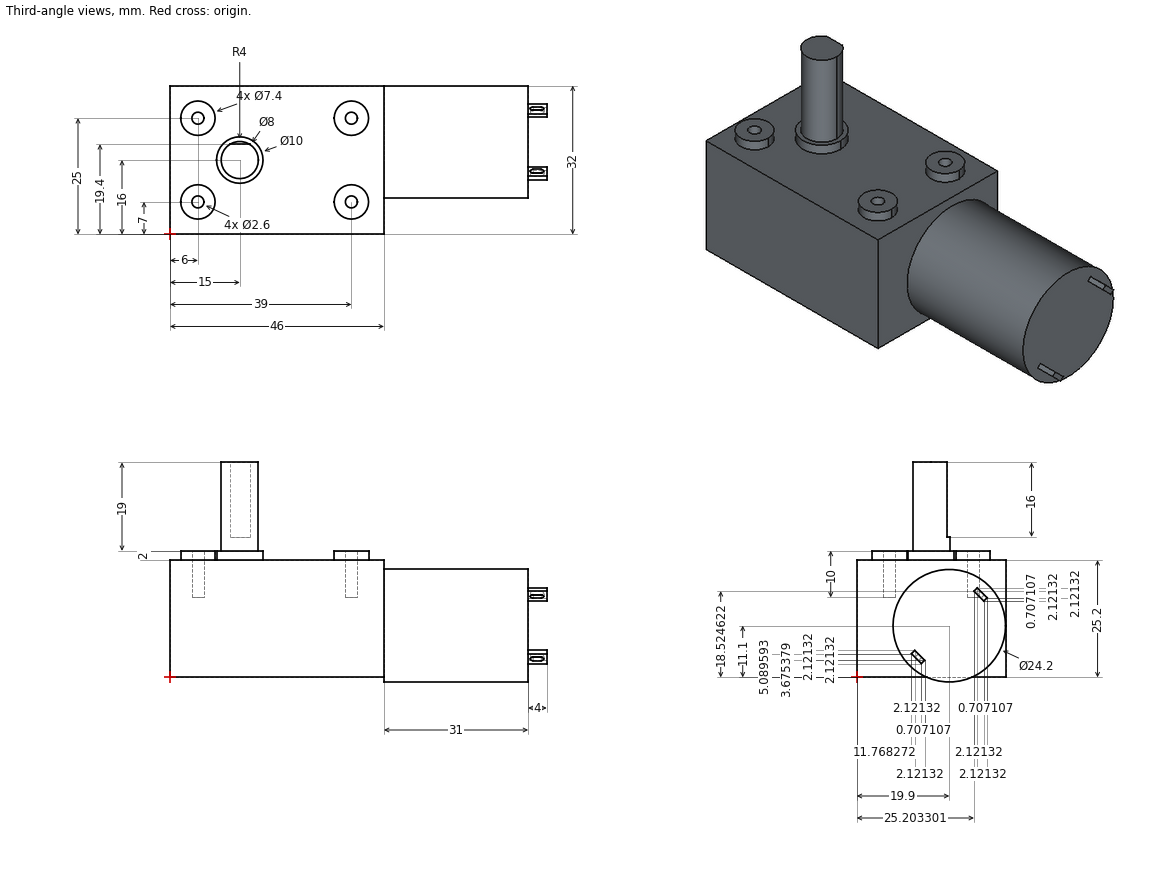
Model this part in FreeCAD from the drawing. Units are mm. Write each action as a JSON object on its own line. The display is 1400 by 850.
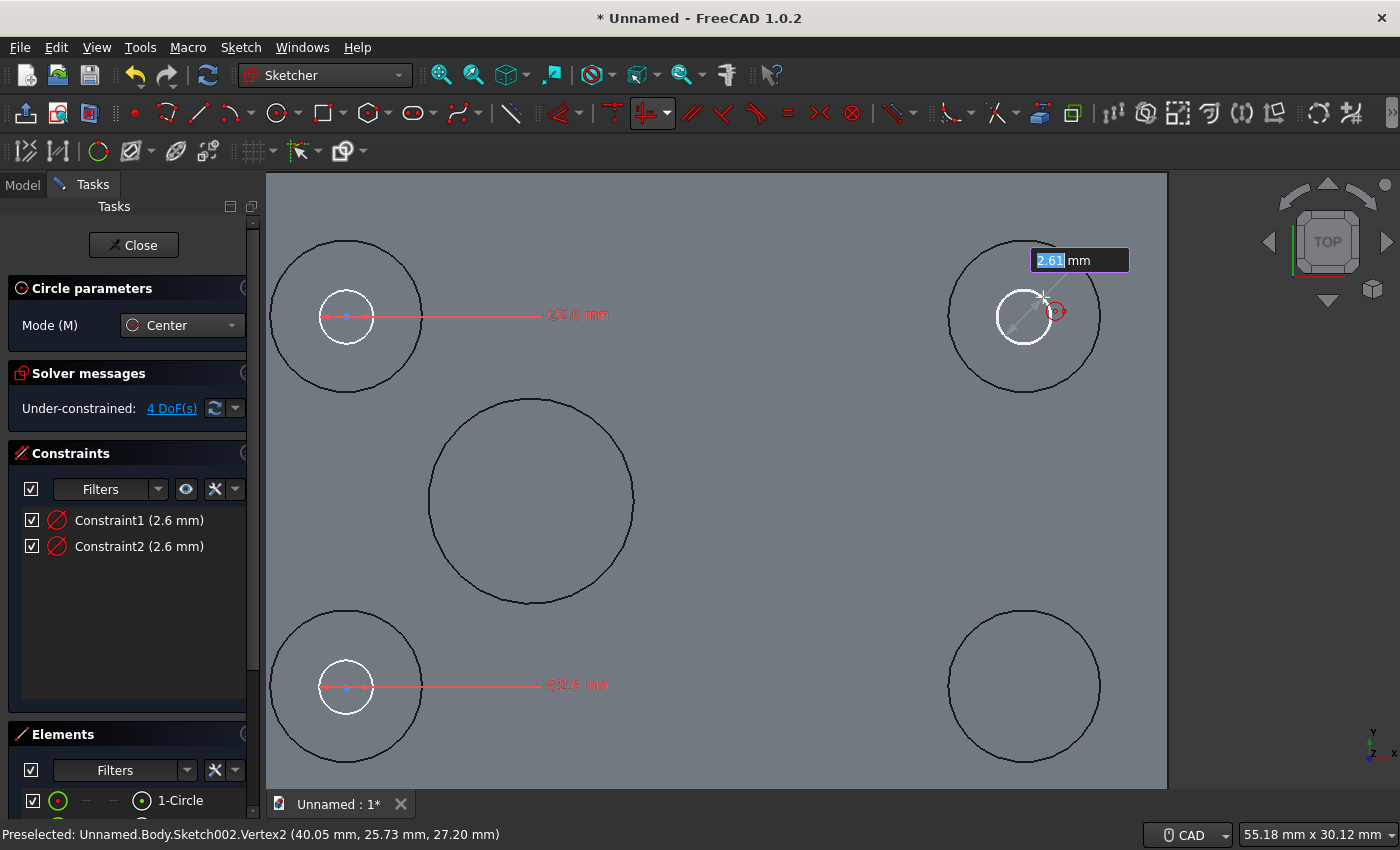
{"action": "type", "text": "2.6"}
{"action": "key", "text": "Return"}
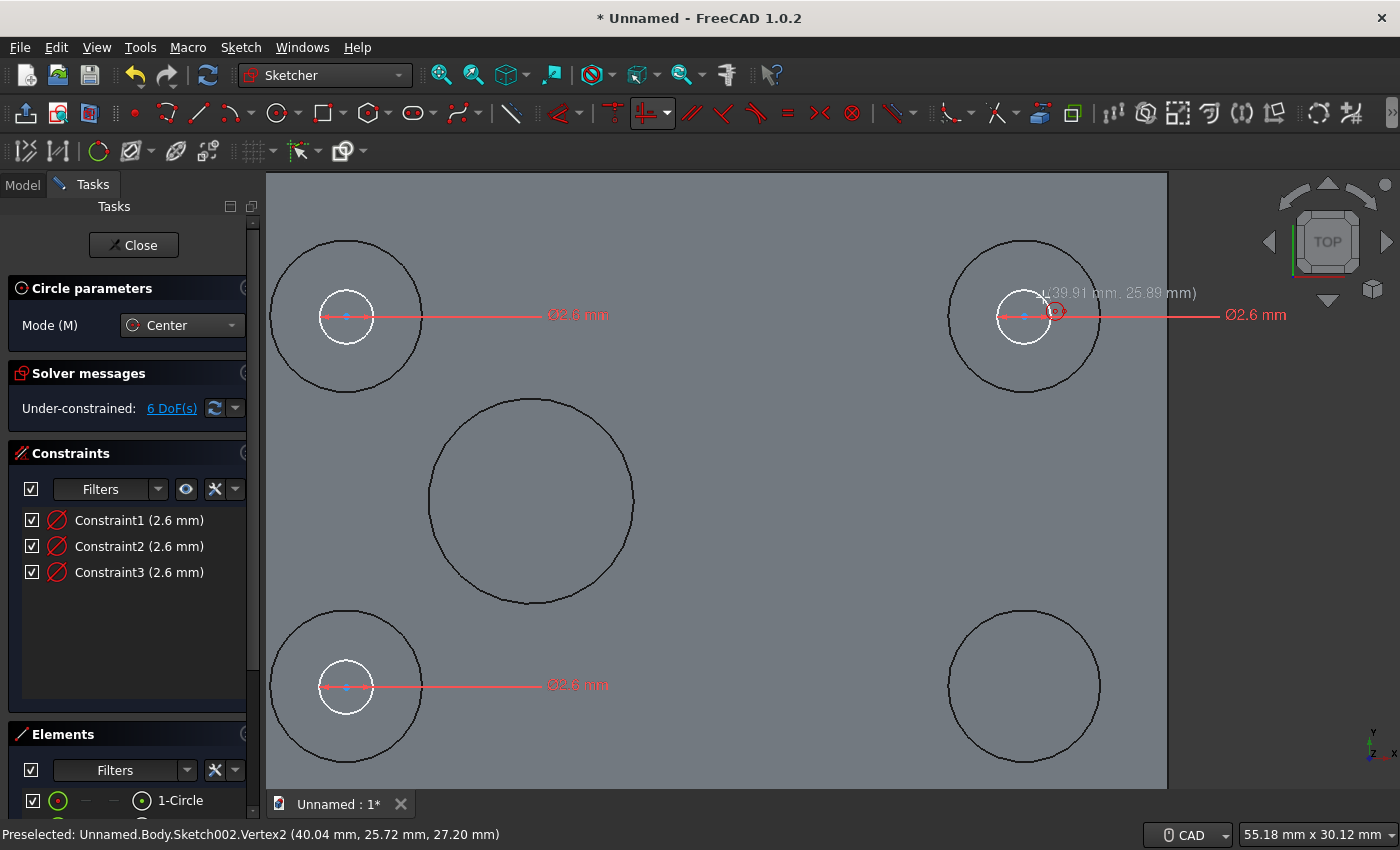
{"action": "left_click", "coordinate": [1024, 686]}
{"action": "mouse_move", "coordinate": [1043, 667]}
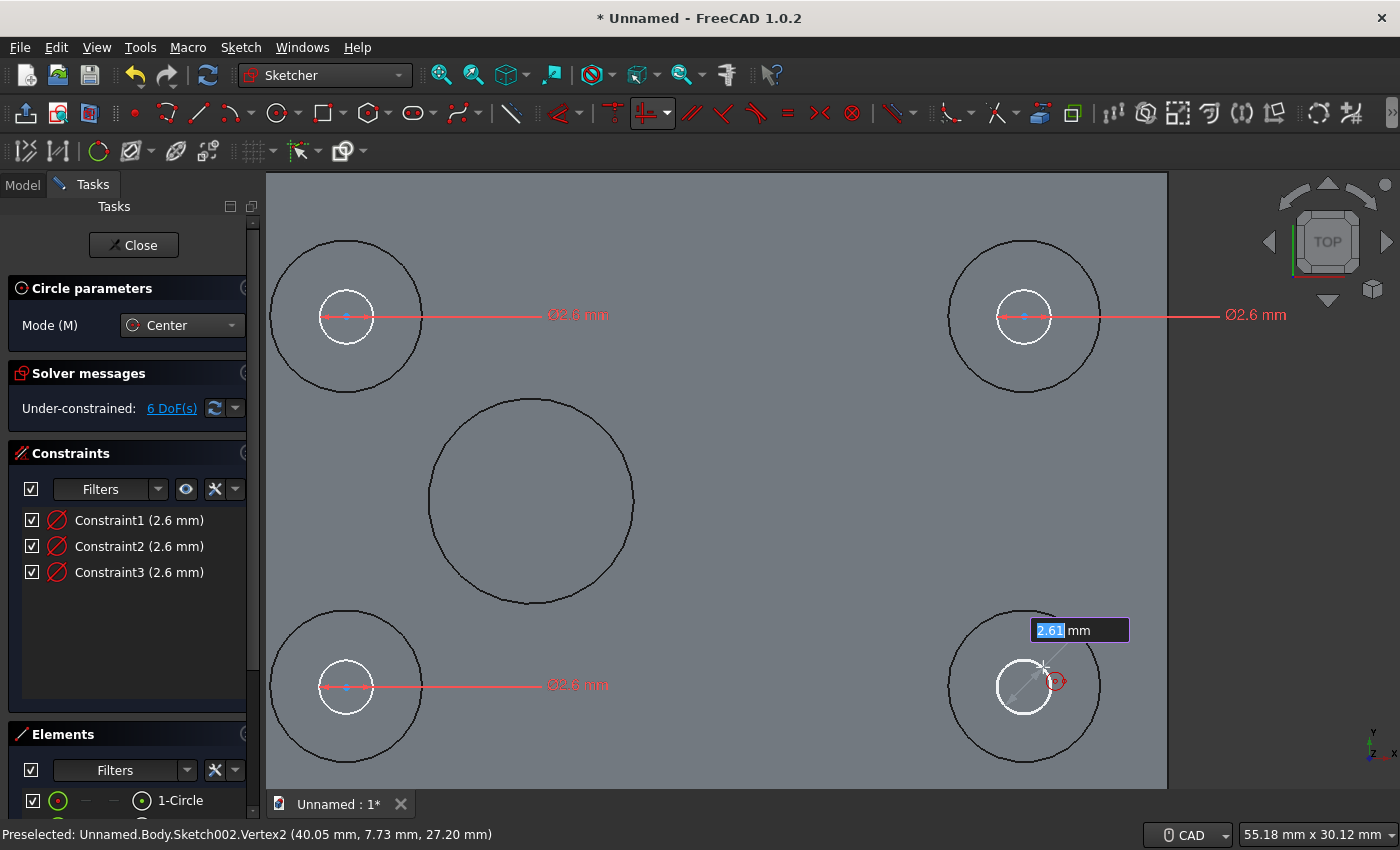
{"action": "type", "text": "2.6"}
{"action": "key", "text": "Return"}
{"action": "key", "text": "Escape"}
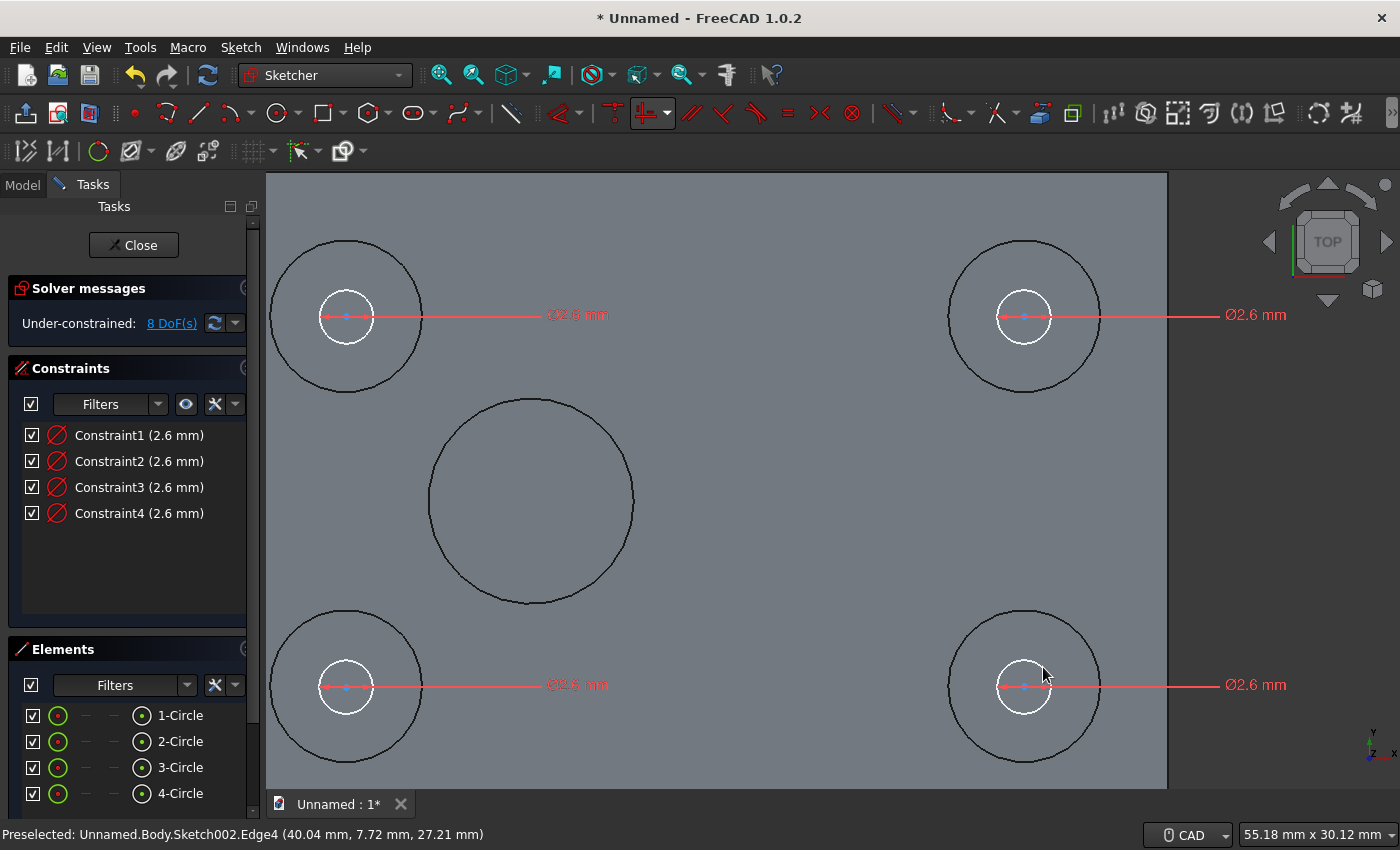
{"action": "left_click", "coordinate": [346, 687]}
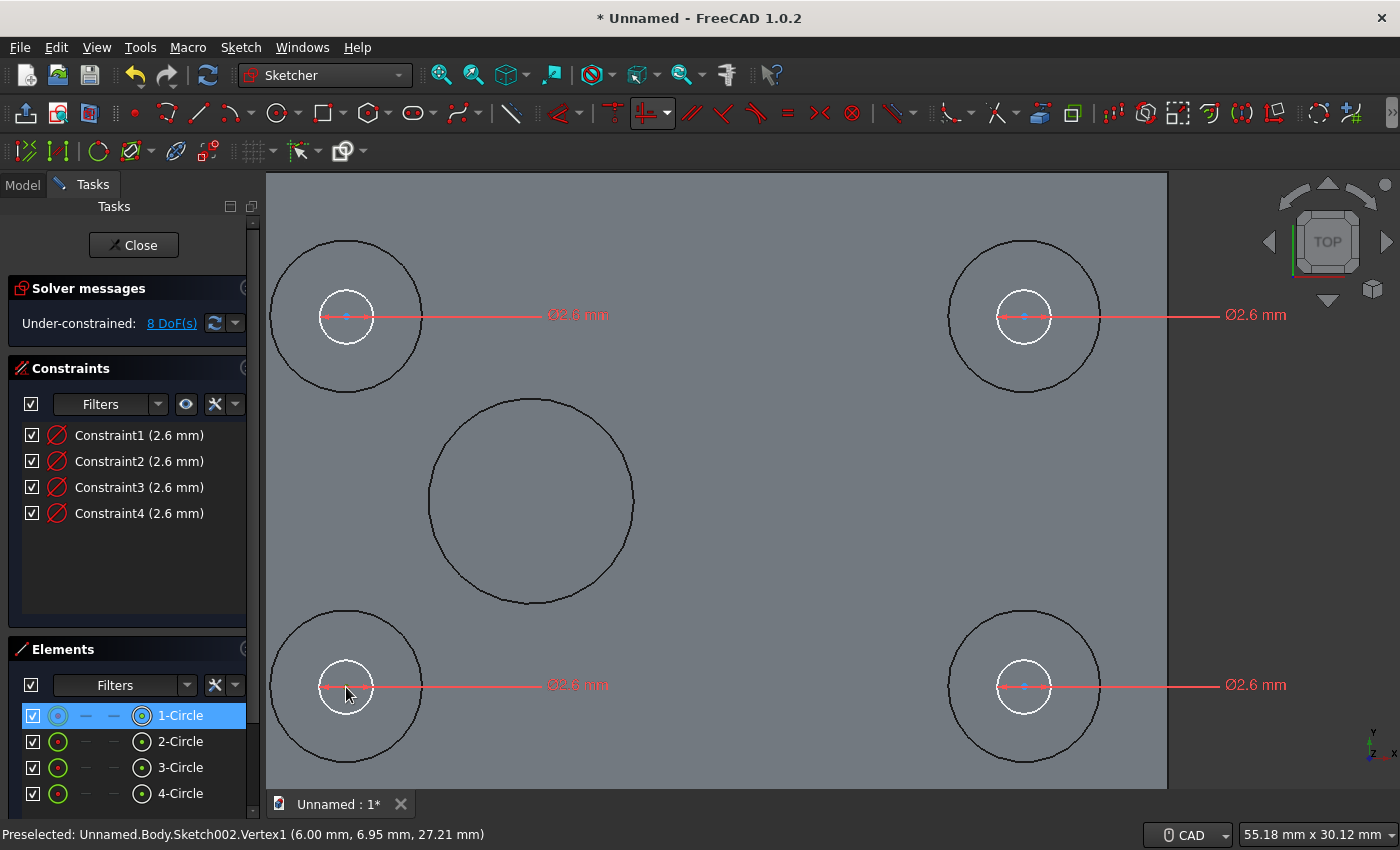
{"action": "left_click", "coordinate": [347, 317]}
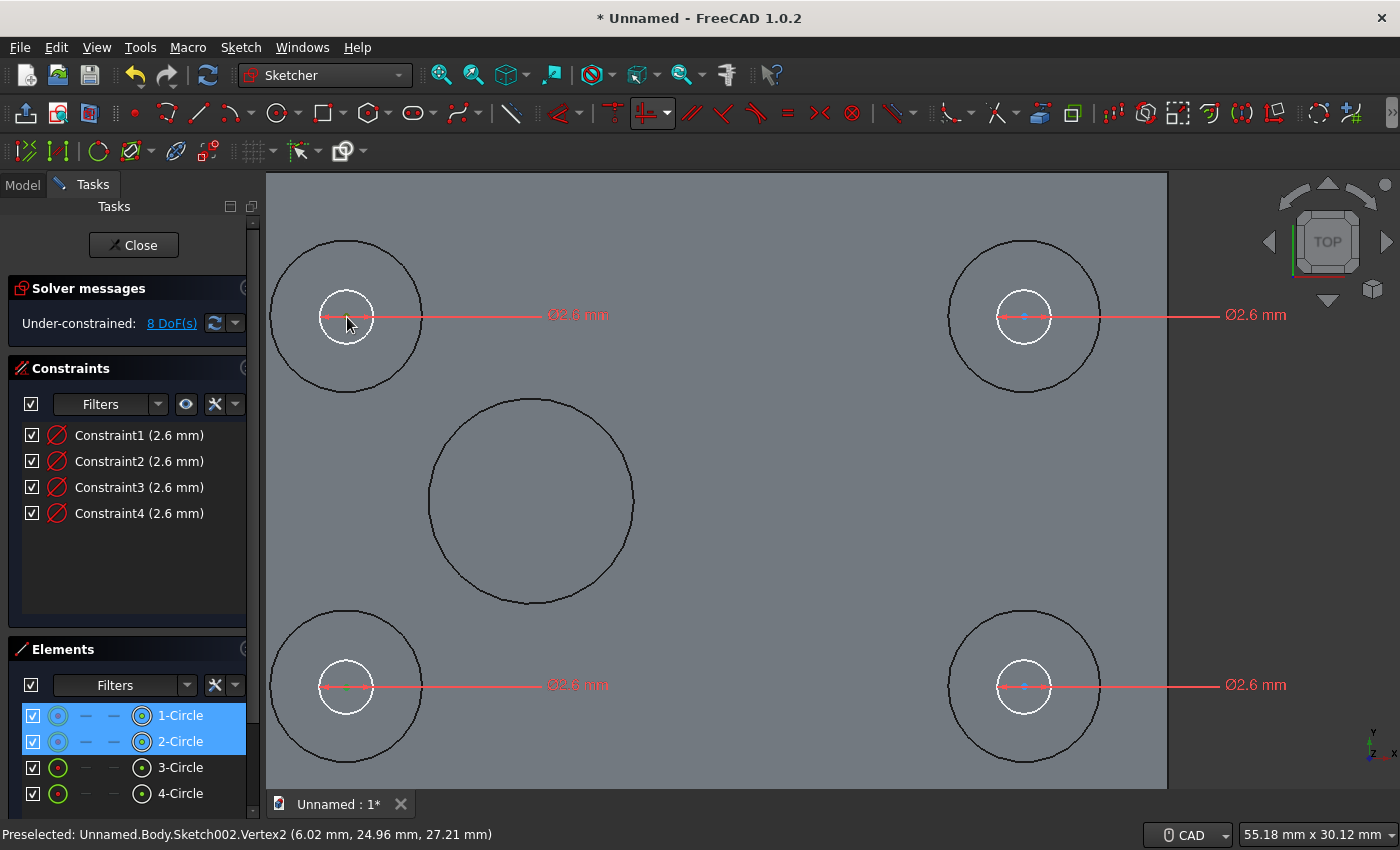
{"action": "left_click", "coordinate": [670, 114]}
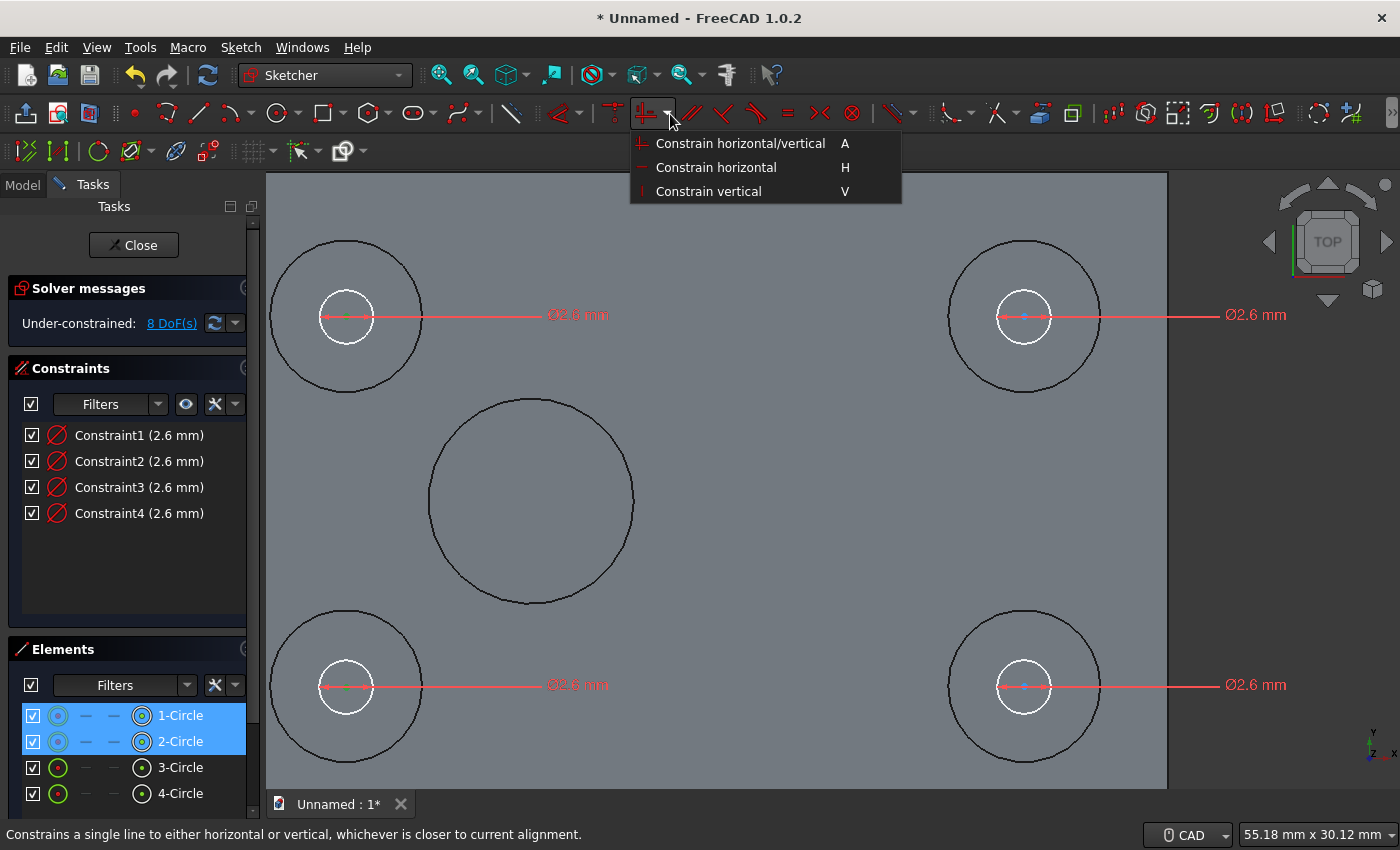
{"action": "left_click", "coordinate": [766, 191]}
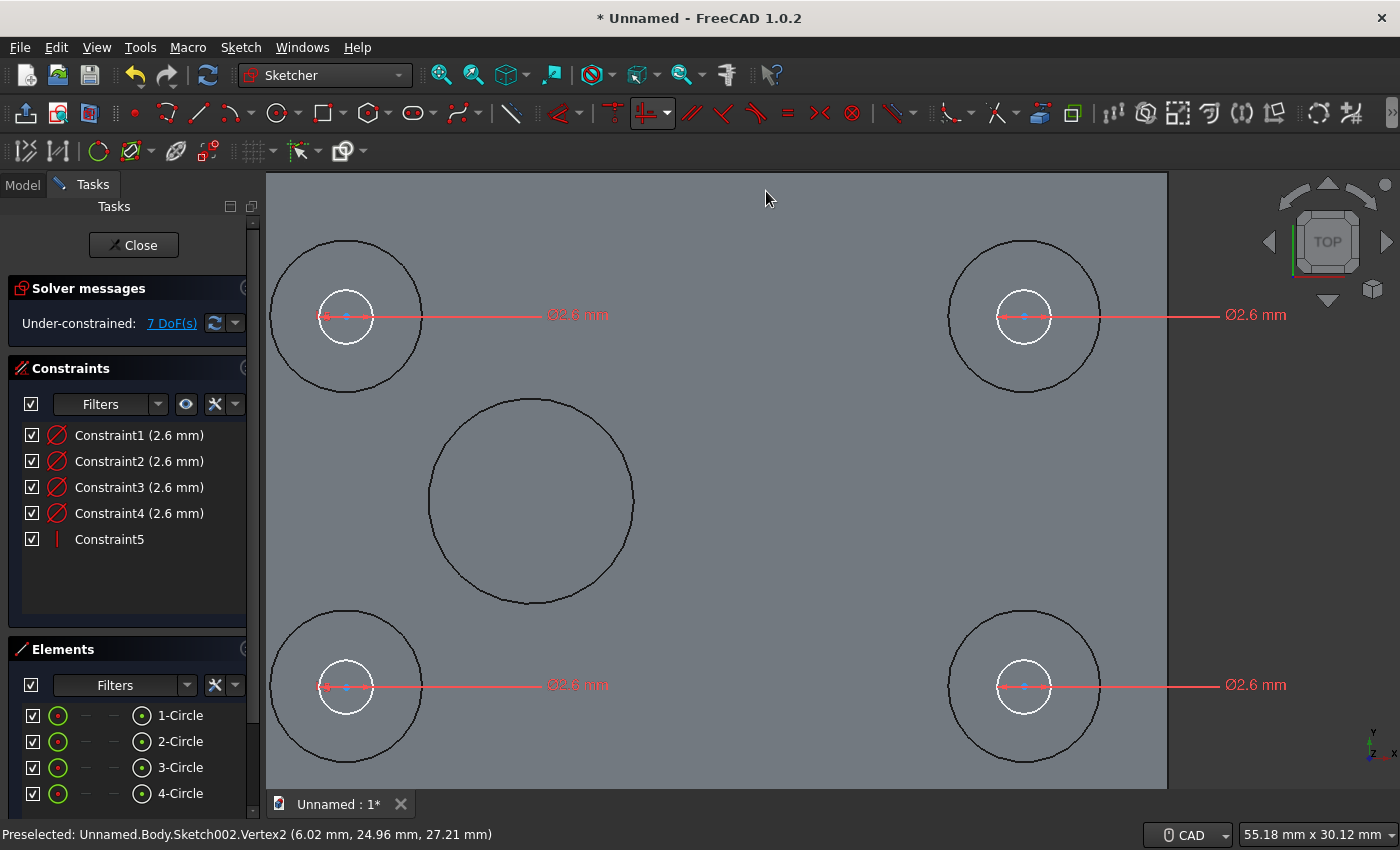
{"action": "left_click", "coordinate": [346, 317]}